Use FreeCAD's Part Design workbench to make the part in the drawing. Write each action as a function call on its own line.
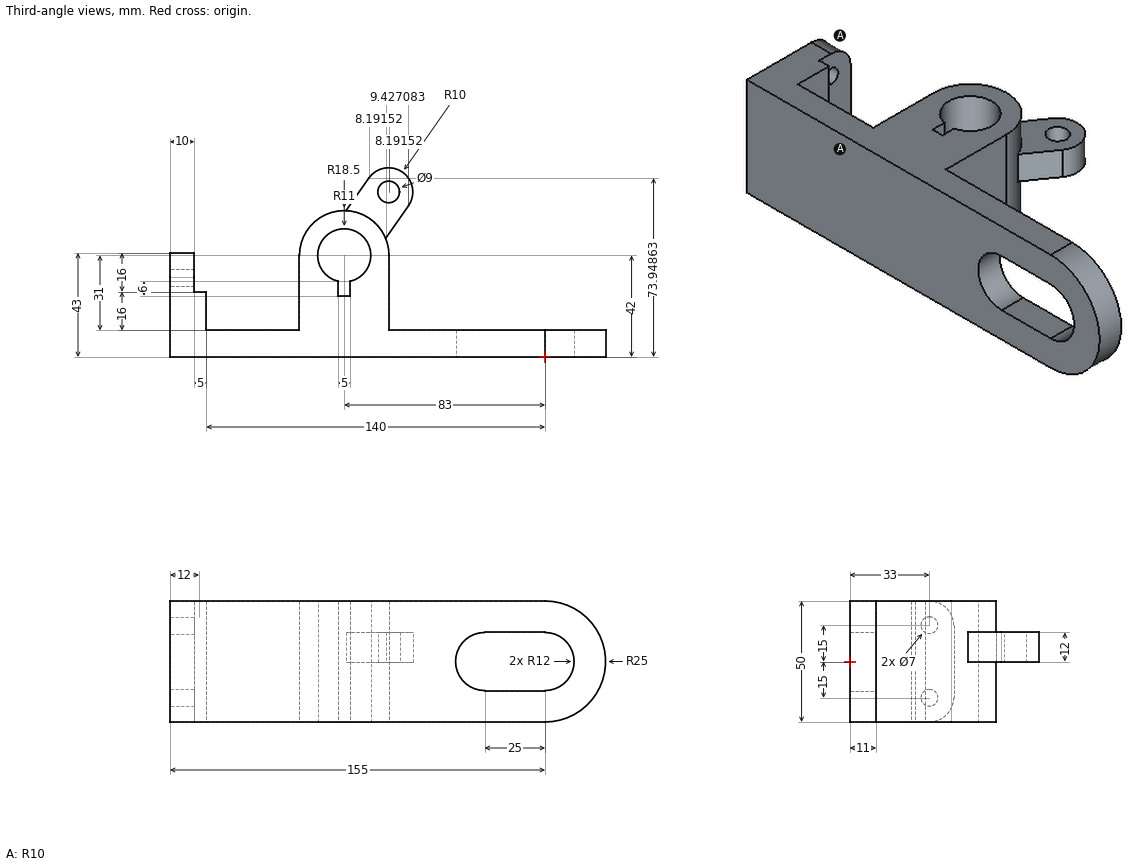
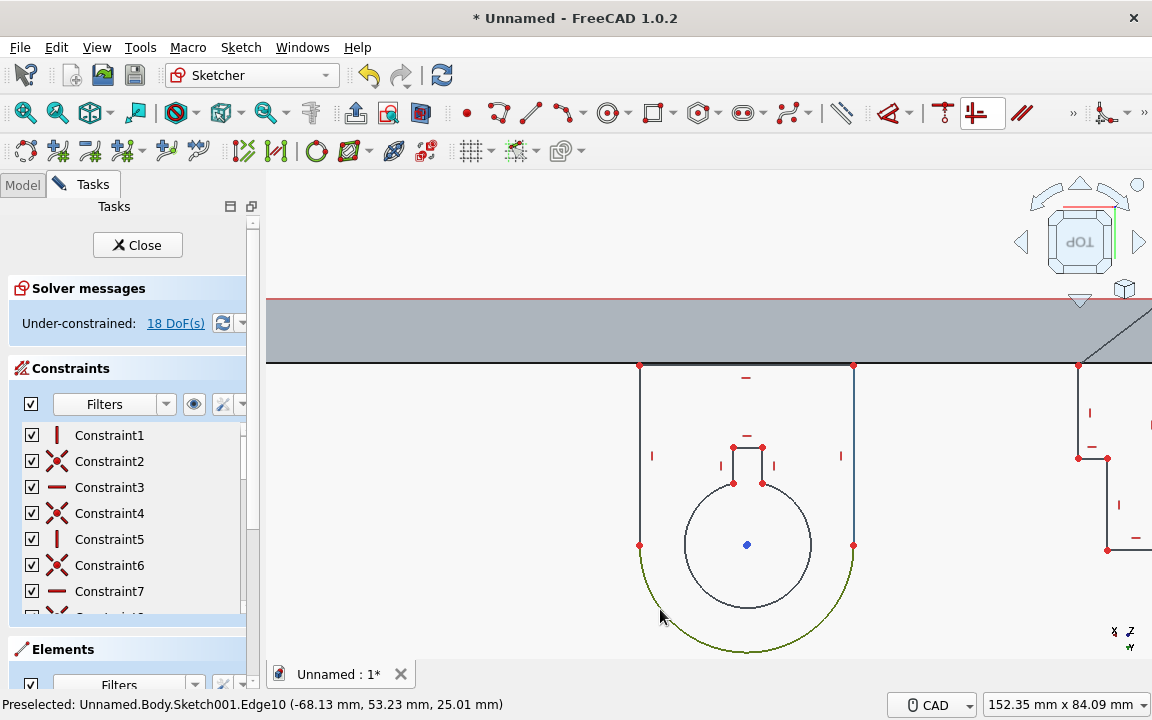
key(t)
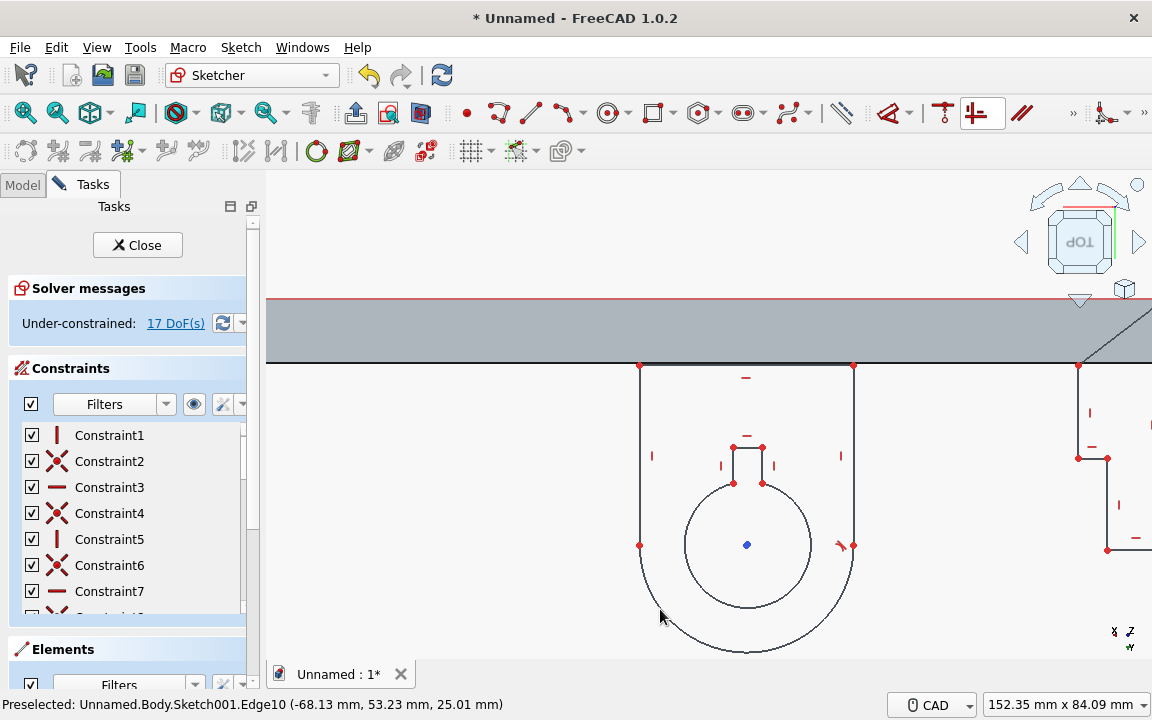
click(640, 420)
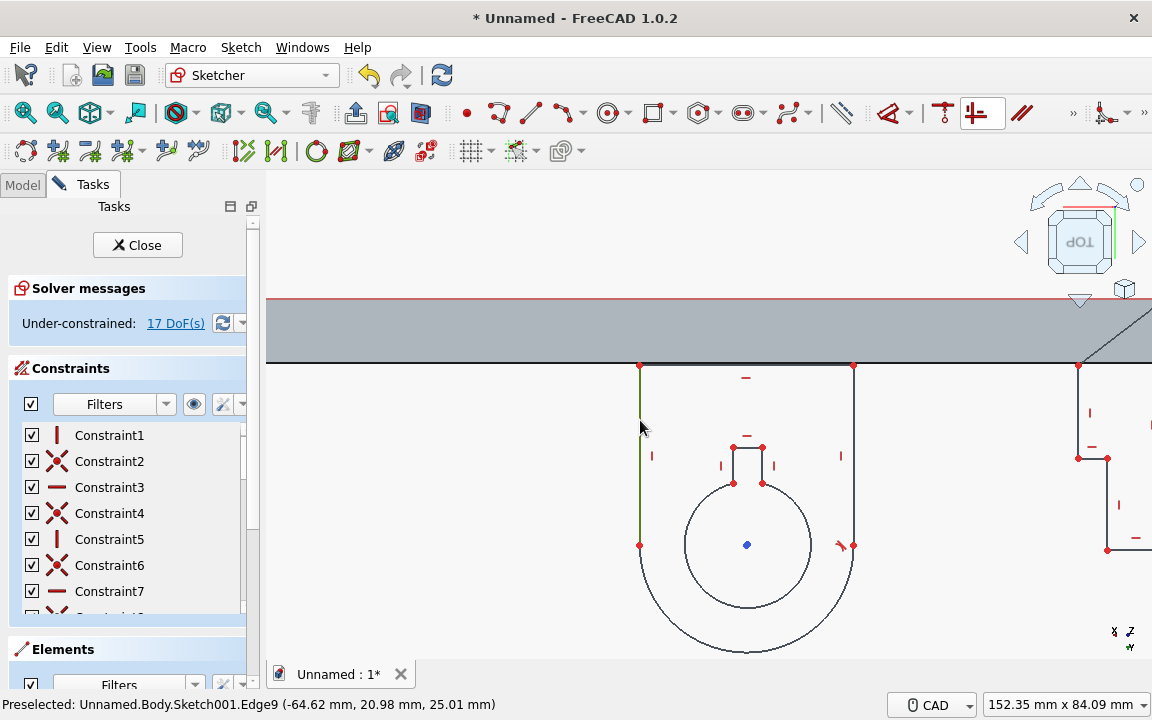
click(660, 609)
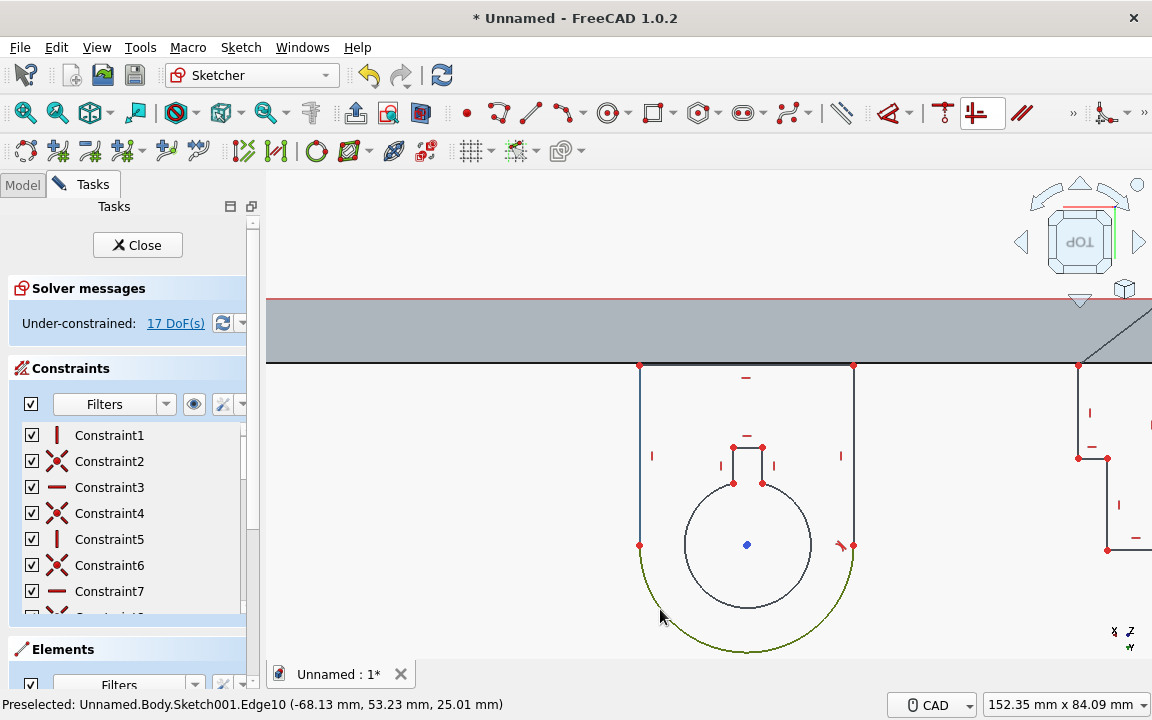
key(t)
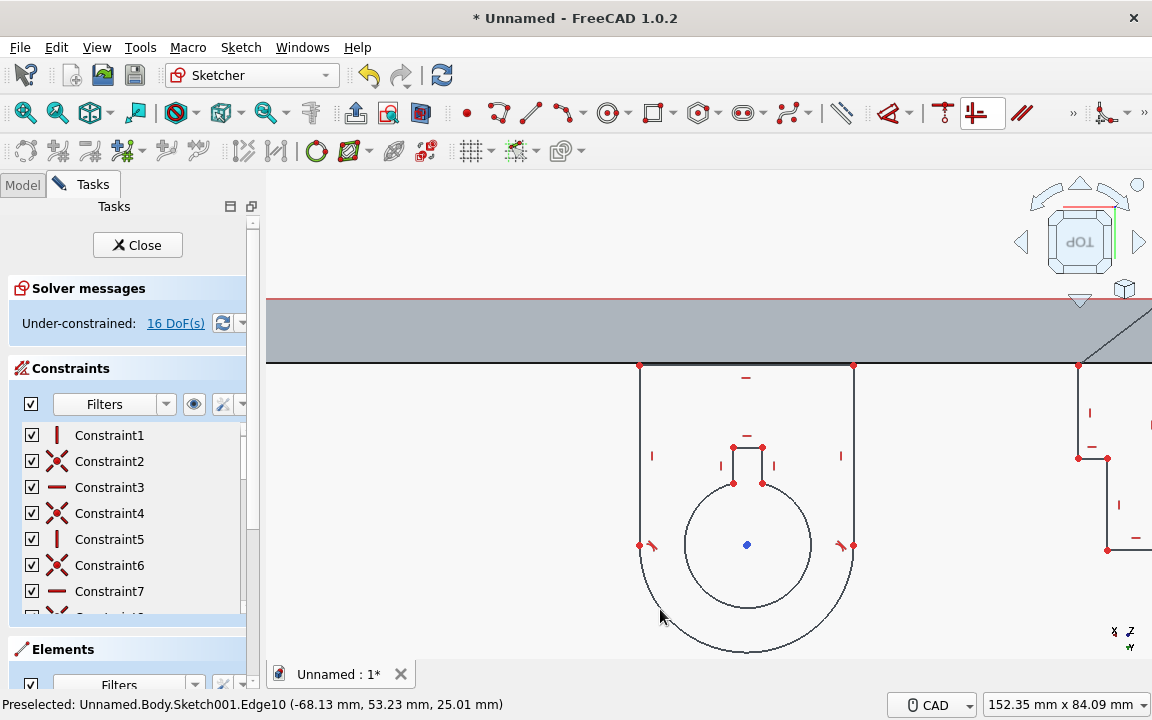
click(660, 609)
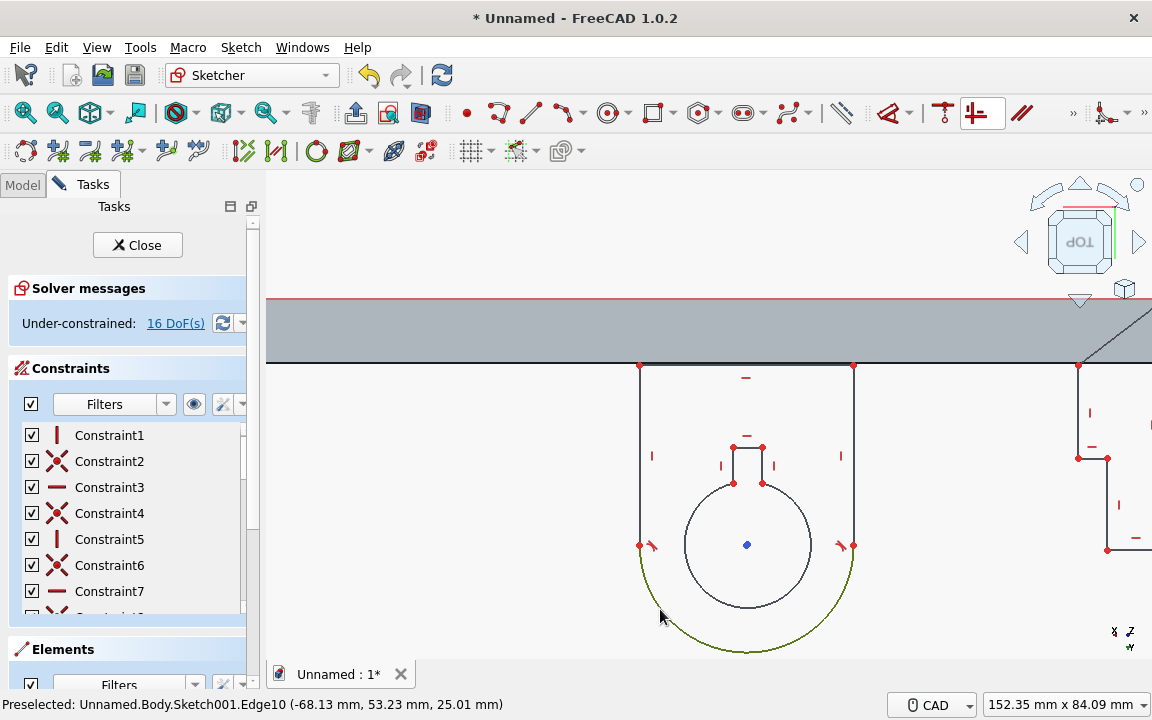
click(690, 570)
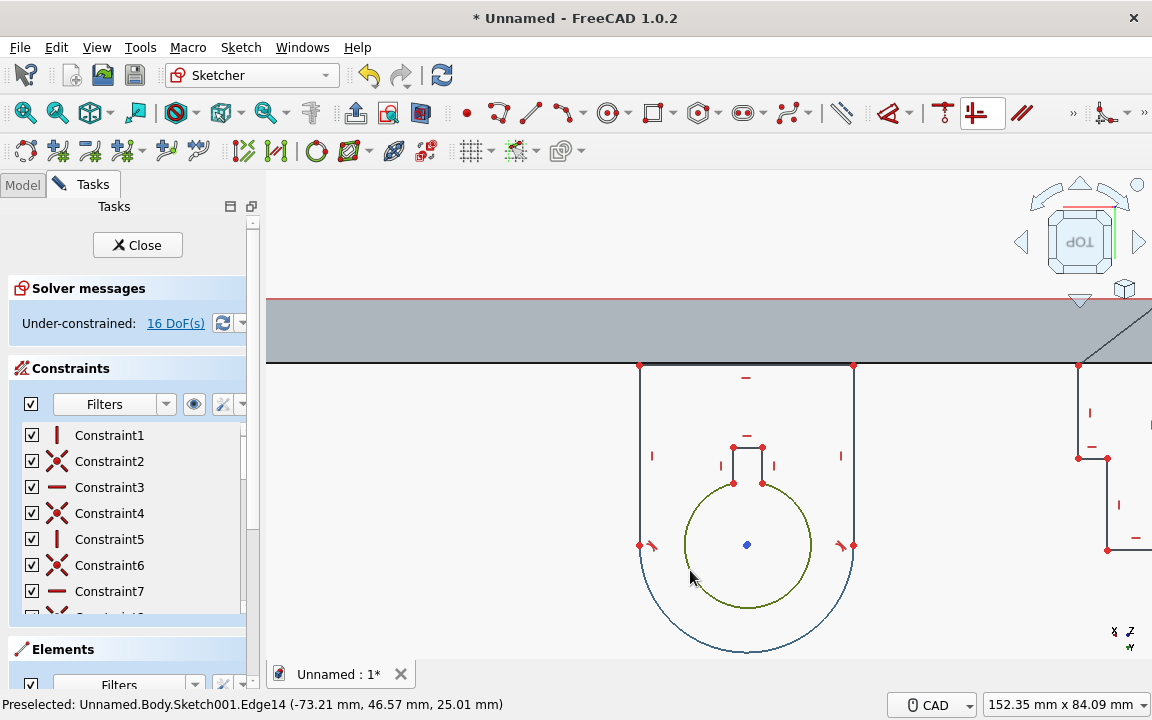
click(944, 114)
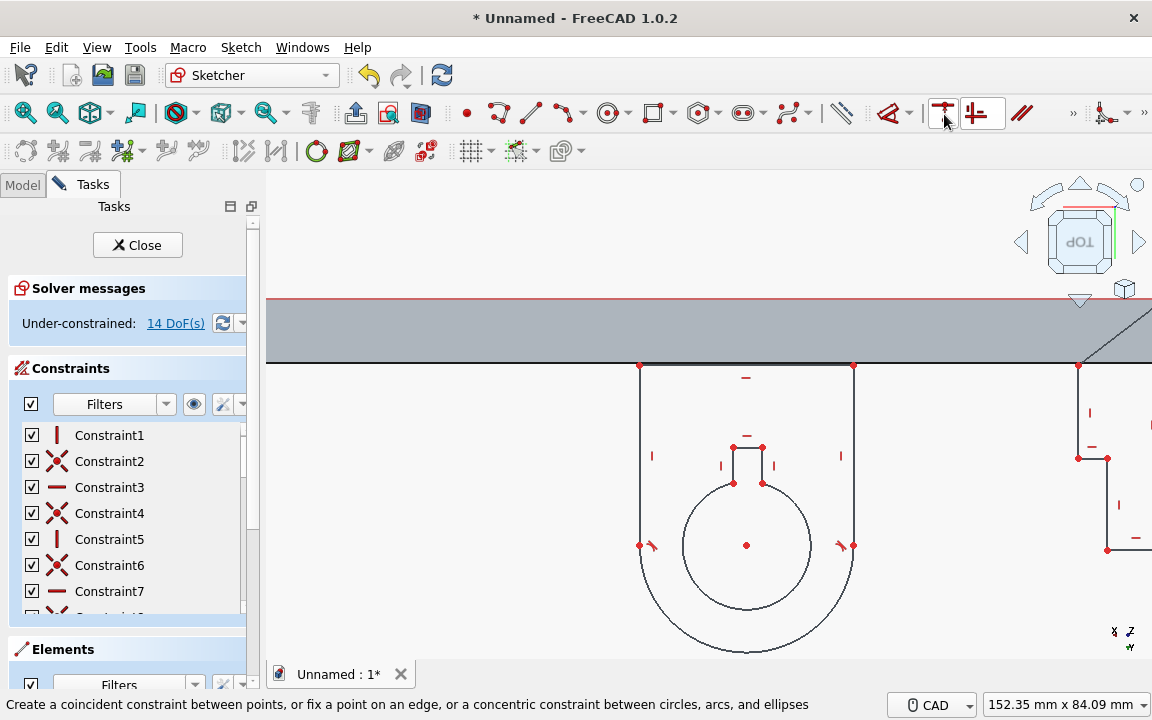
click(888, 114)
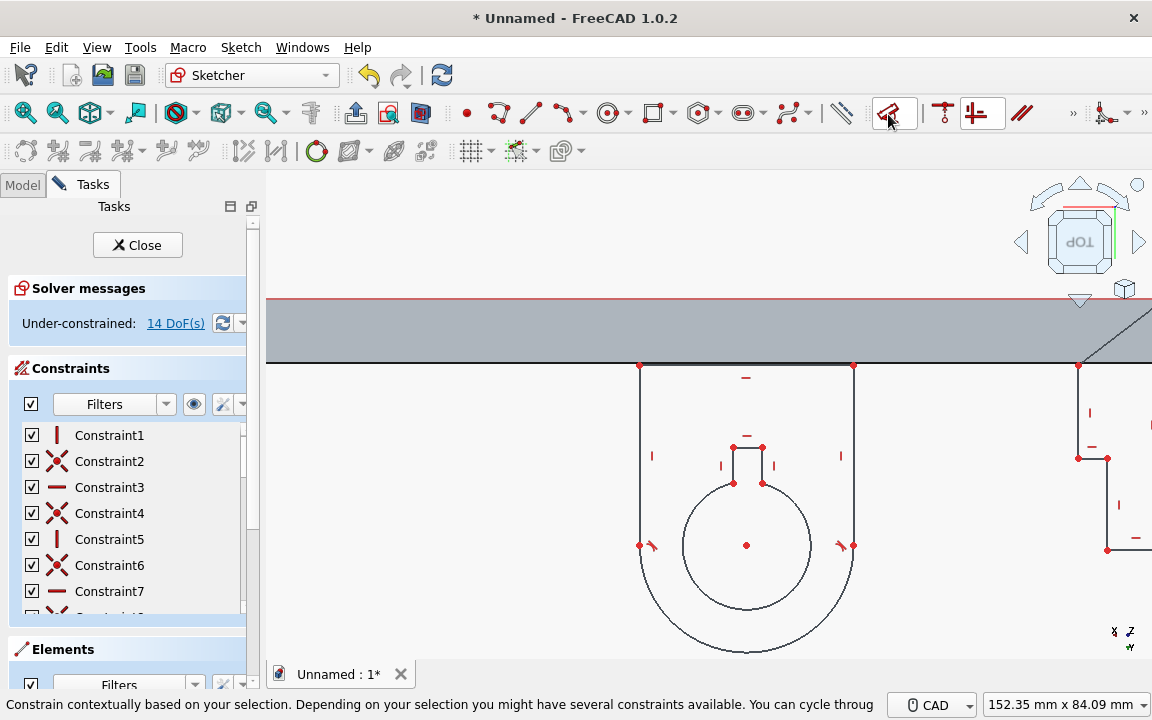
click(660, 609)
click(634, 628)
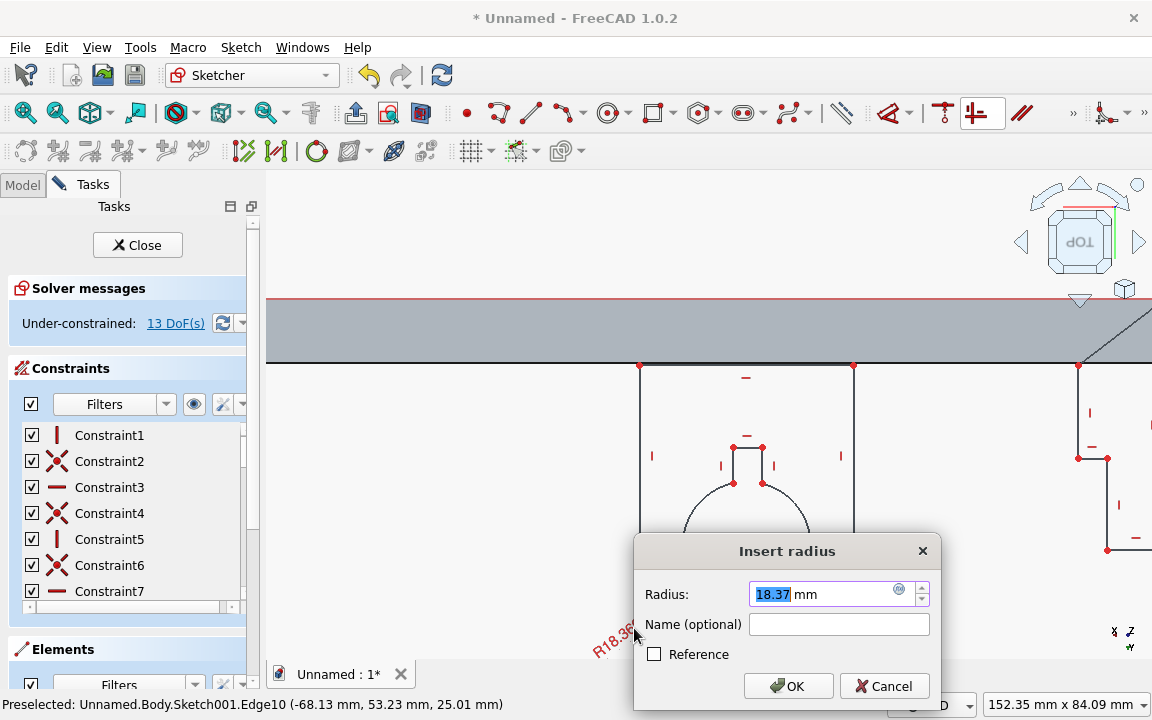
text(18.5)
key(Return)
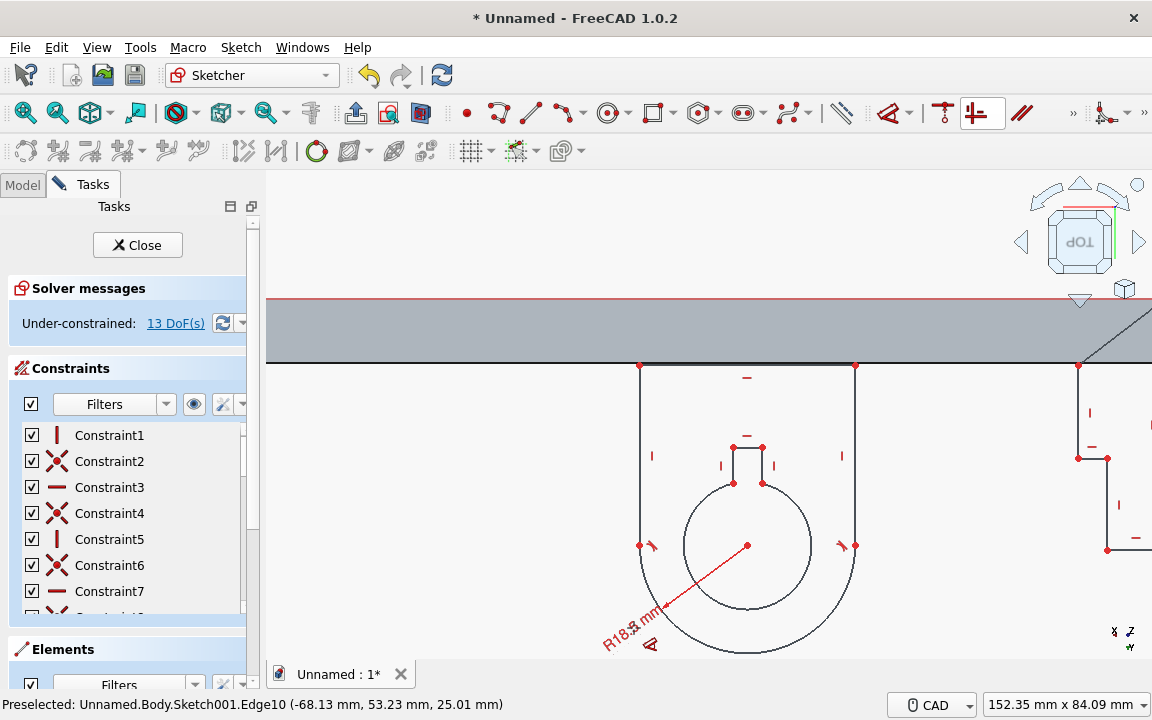
click(689, 571)
click(668, 492)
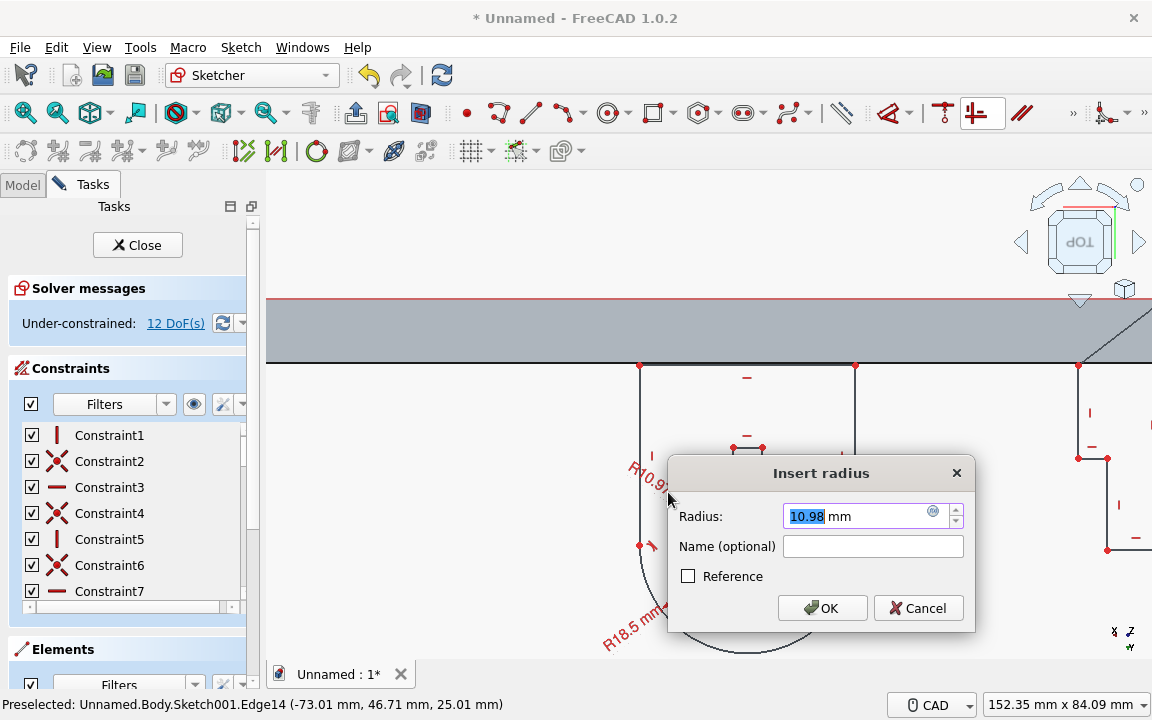
text(11)
key(Return)